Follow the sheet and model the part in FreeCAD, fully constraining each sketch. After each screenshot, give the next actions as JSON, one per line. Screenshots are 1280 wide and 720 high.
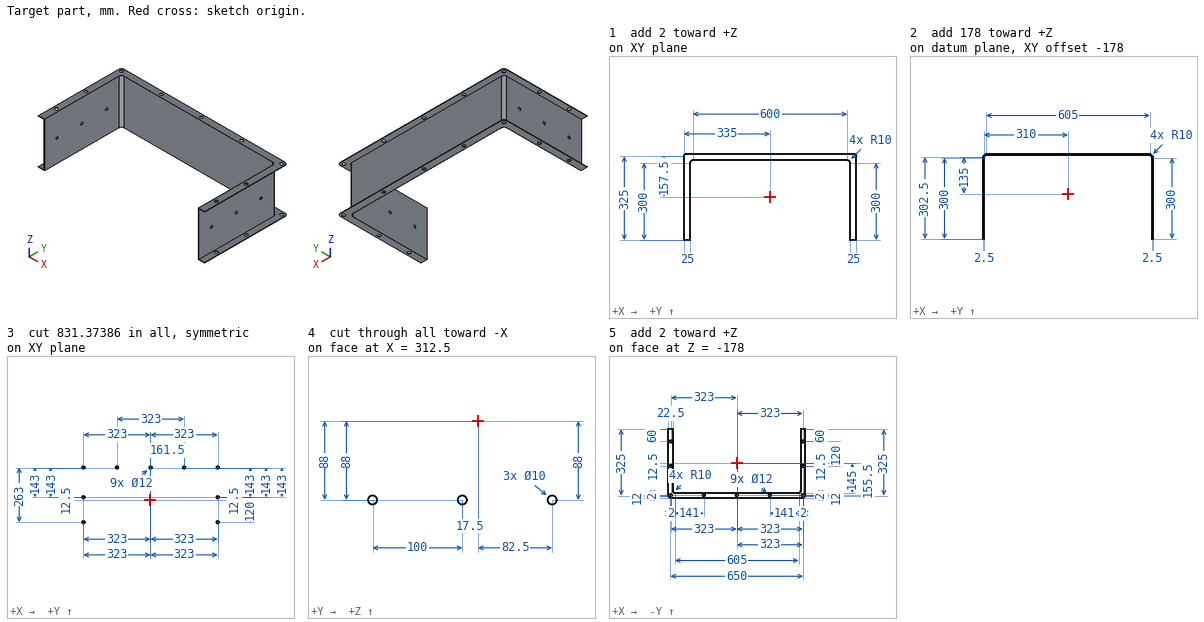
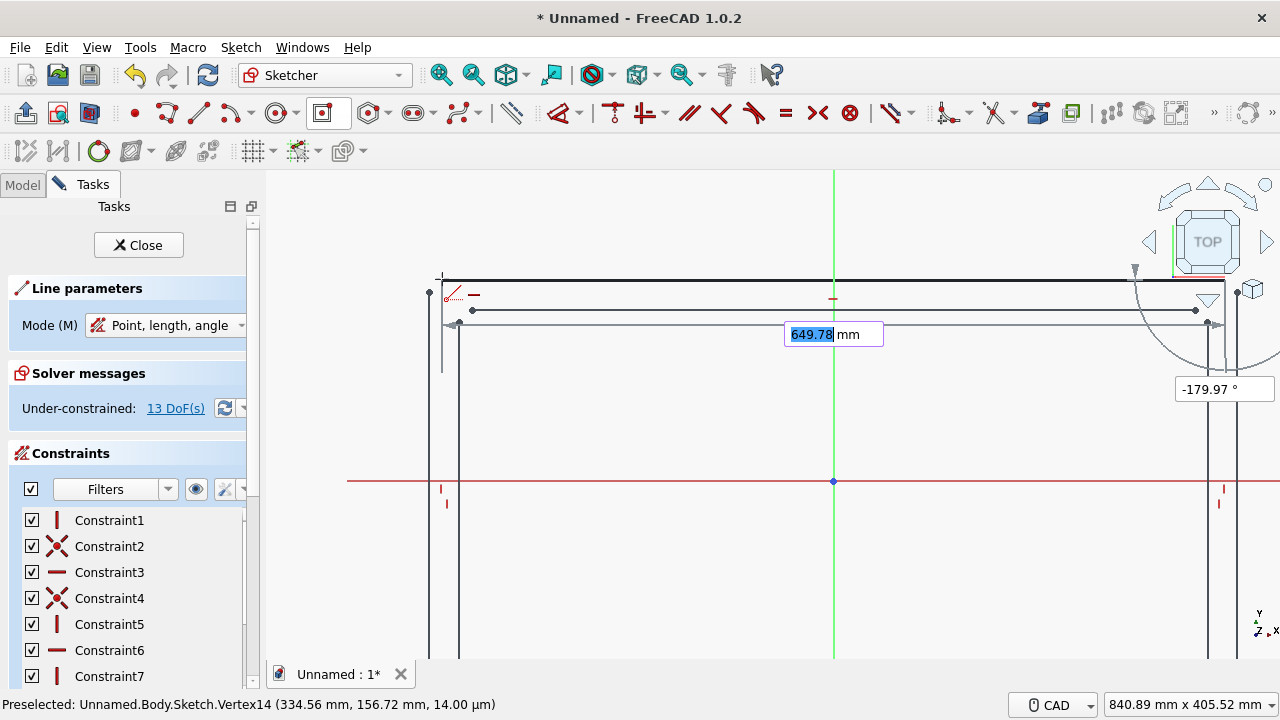
{"action": "left_click", "coordinate": [442, 279]}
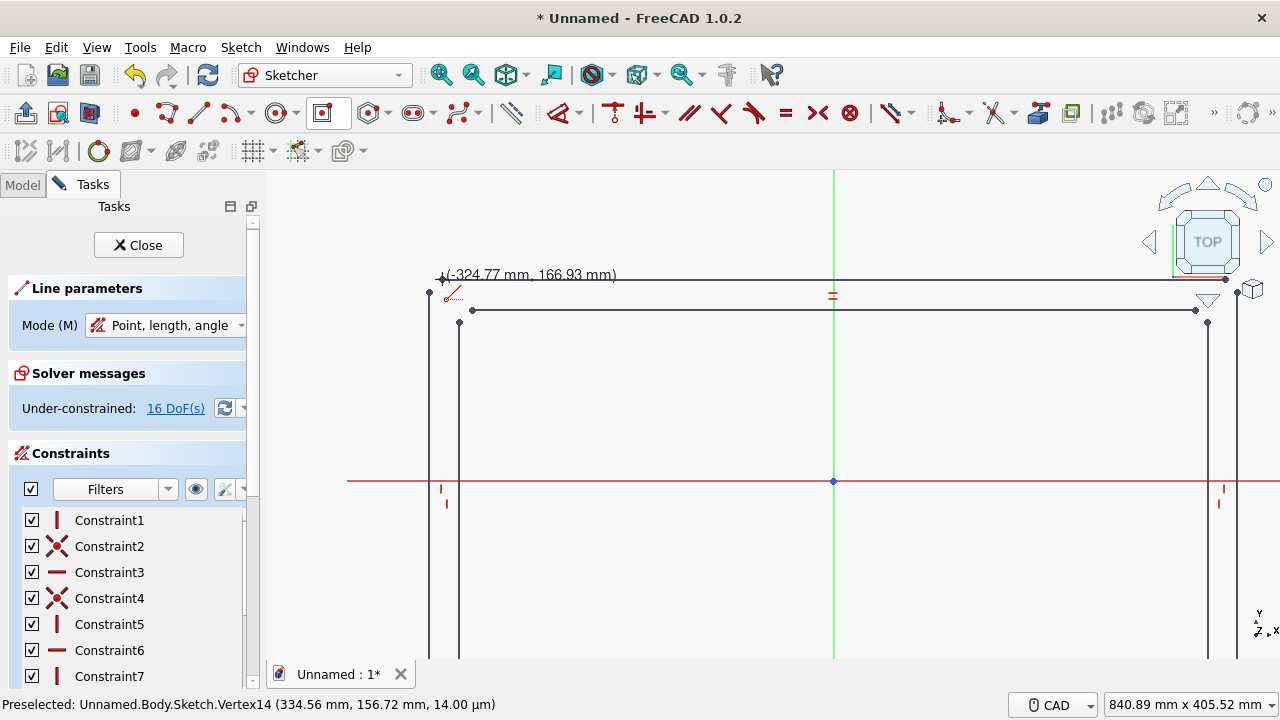
{"action": "left_click", "coordinate": [254, 114]}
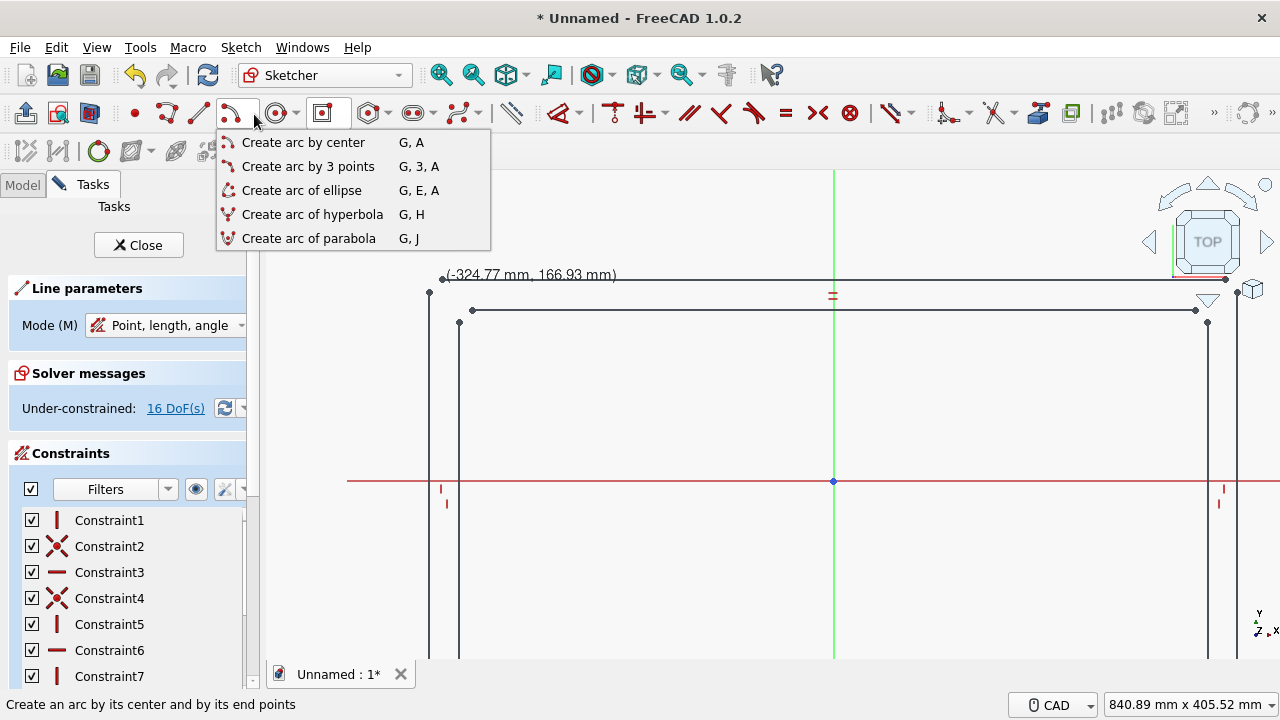
{"action": "left_click", "coordinate": [354, 166]}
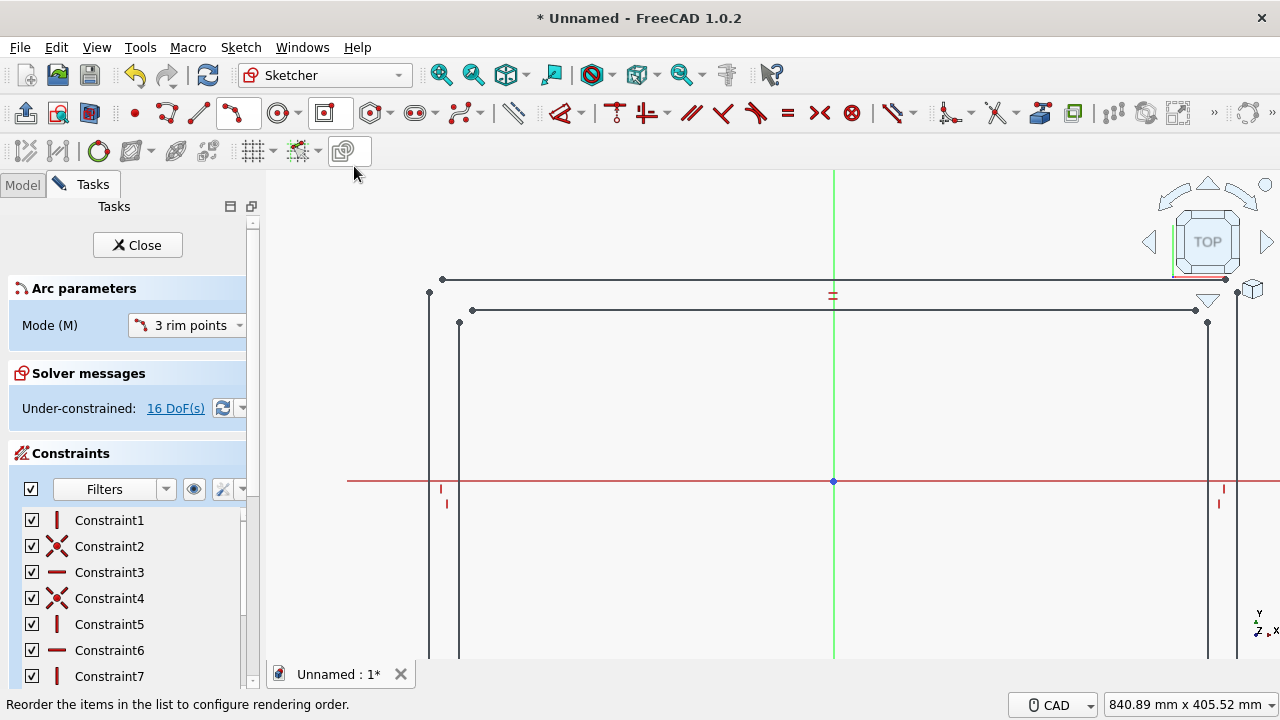
{"action": "left_click", "coordinate": [459, 323]}
{"action": "left_click", "coordinate": [472, 310]}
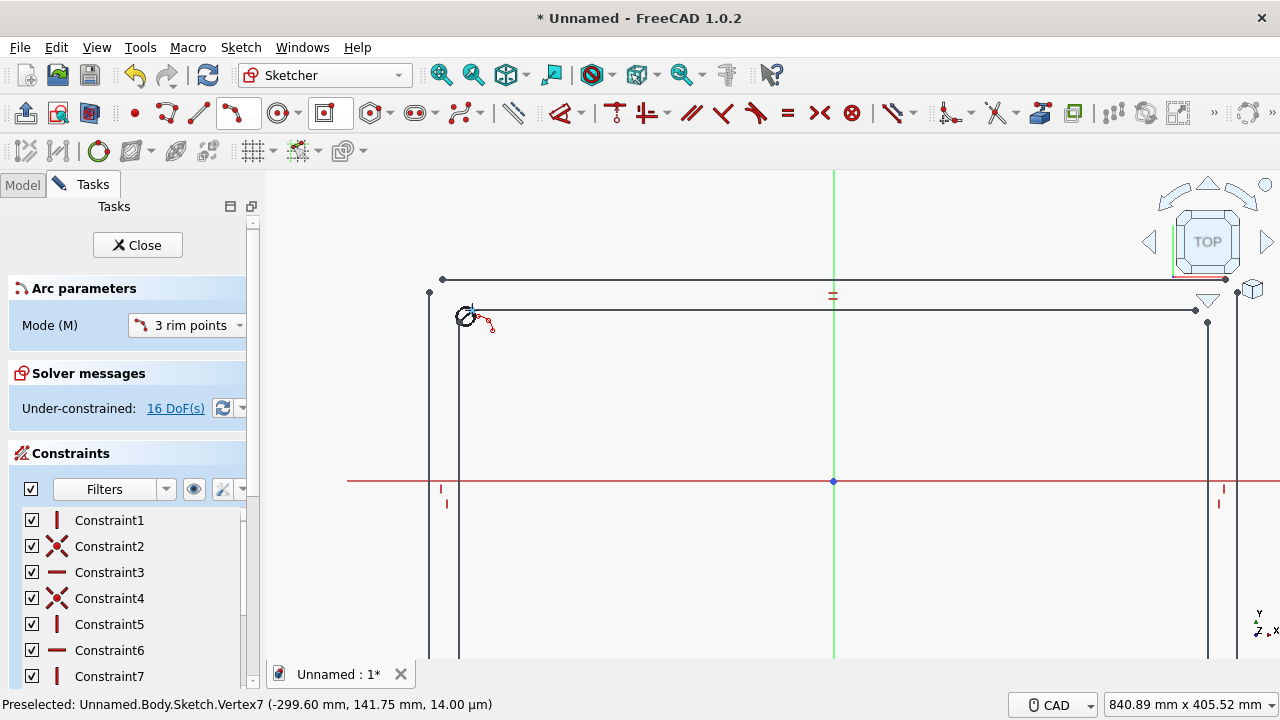
{"action": "scroll", "coordinate": [463, 313], "scroll_direction": "up", "scroll_amount": 8}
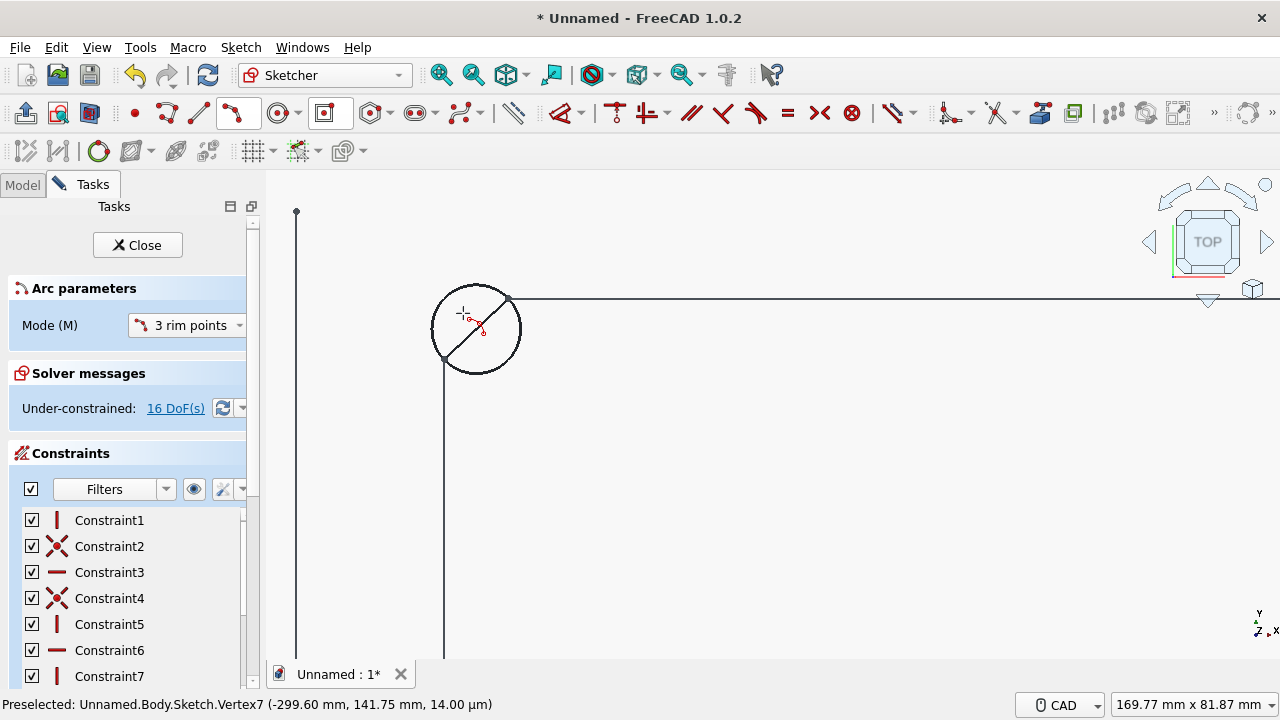
{"action": "left_click", "coordinate": [464, 312]}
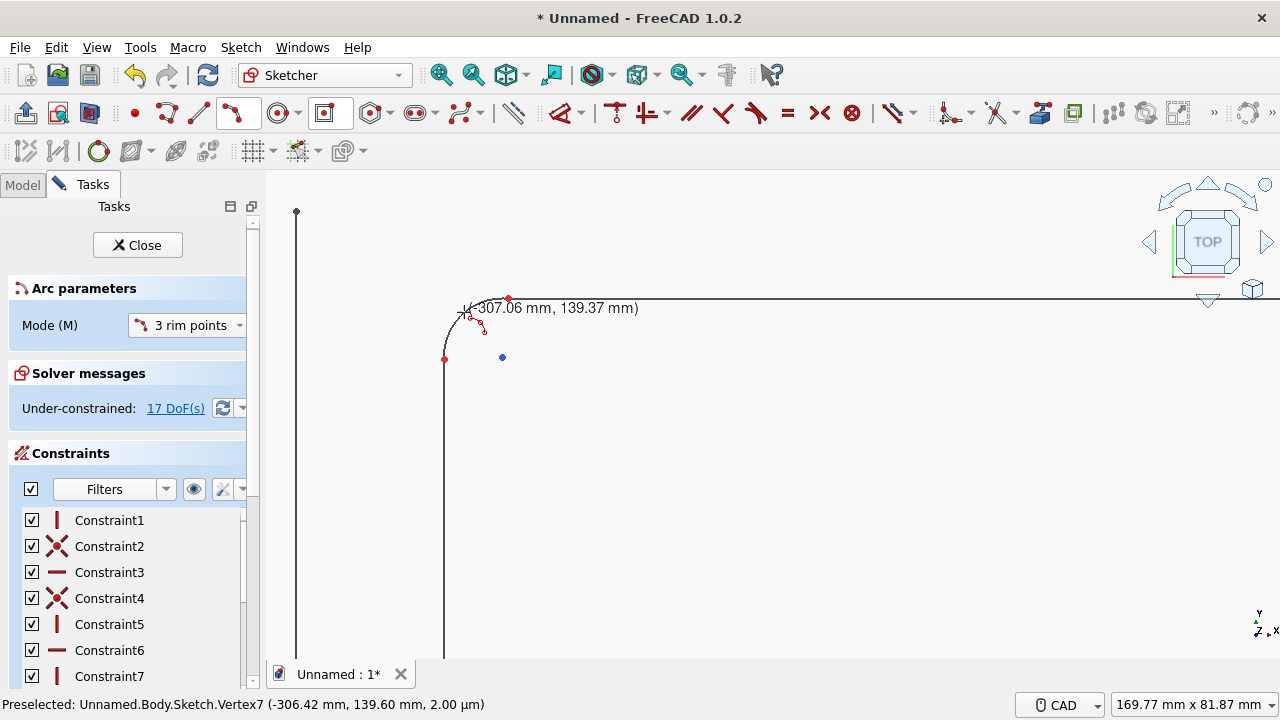
{"action": "scroll", "coordinate": [455, 300], "scroll_direction": "down", "scroll_amount": 10}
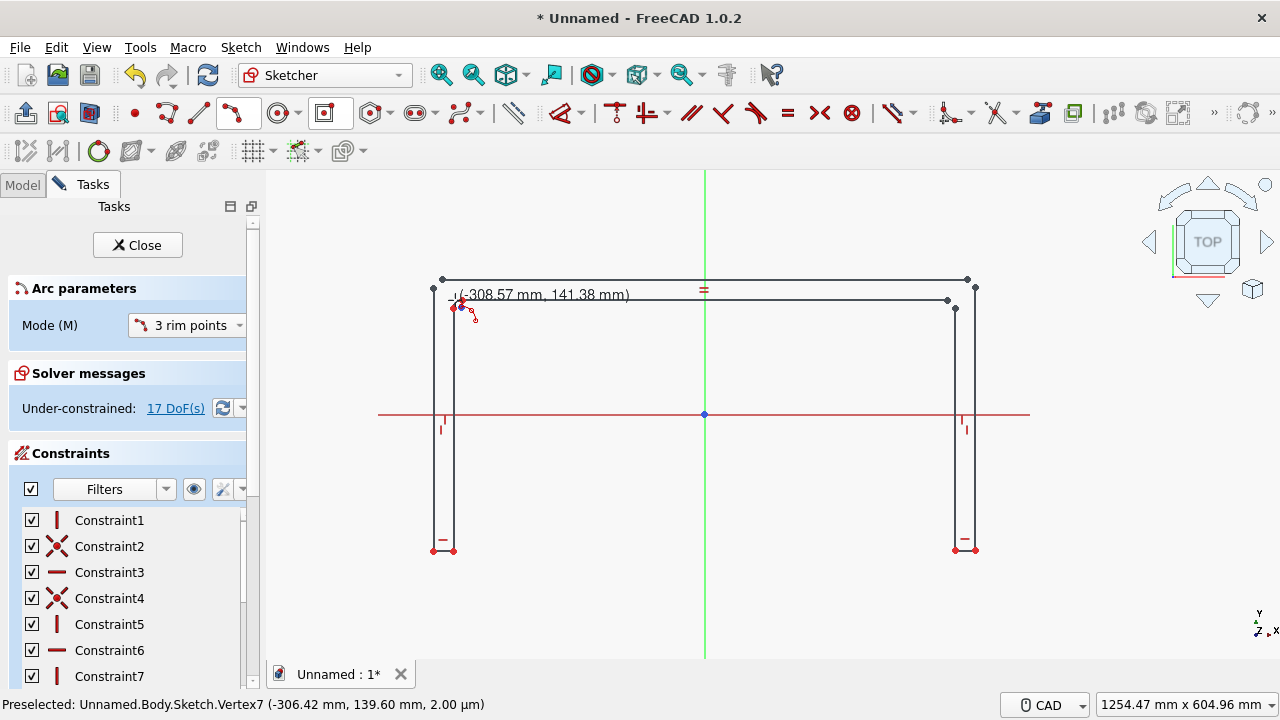
{"action": "scroll", "coordinate": [947, 299], "scroll_direction": "up", "scroll_amount": 2}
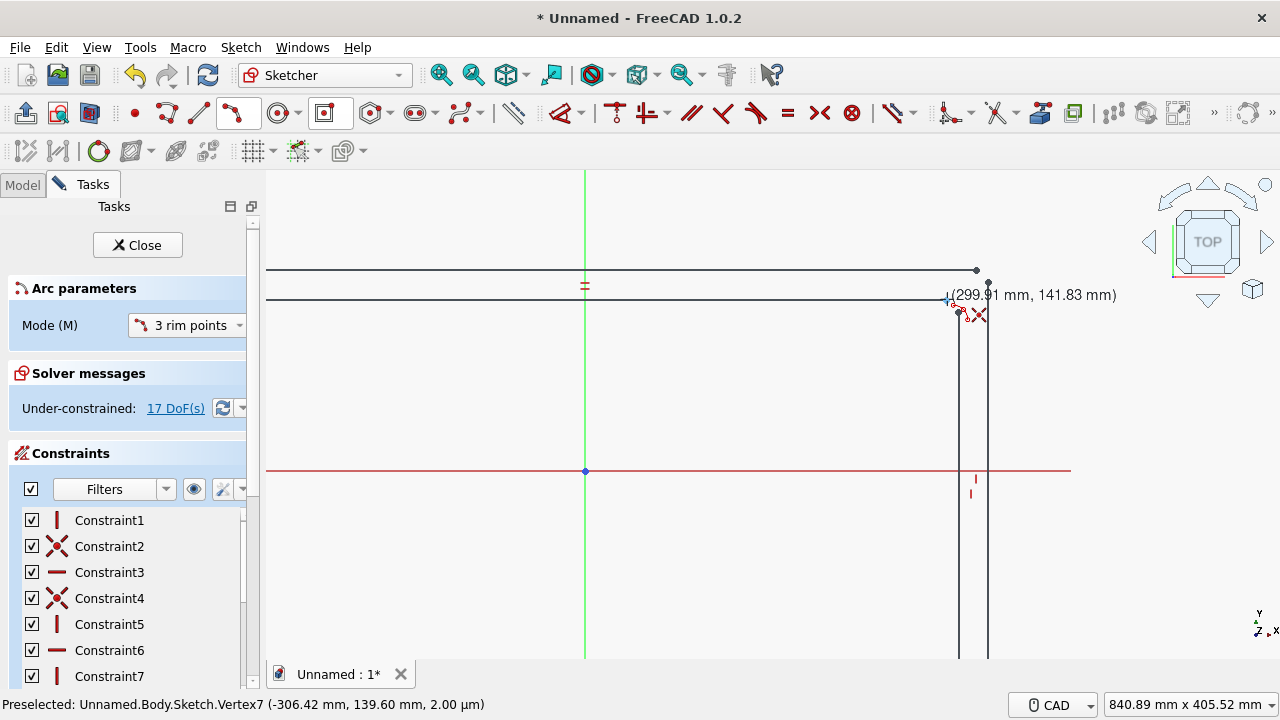
{"action": "left_click", "coordinate": [947, 300]}
{"action": "left_click", "coordinate": [959, 312]}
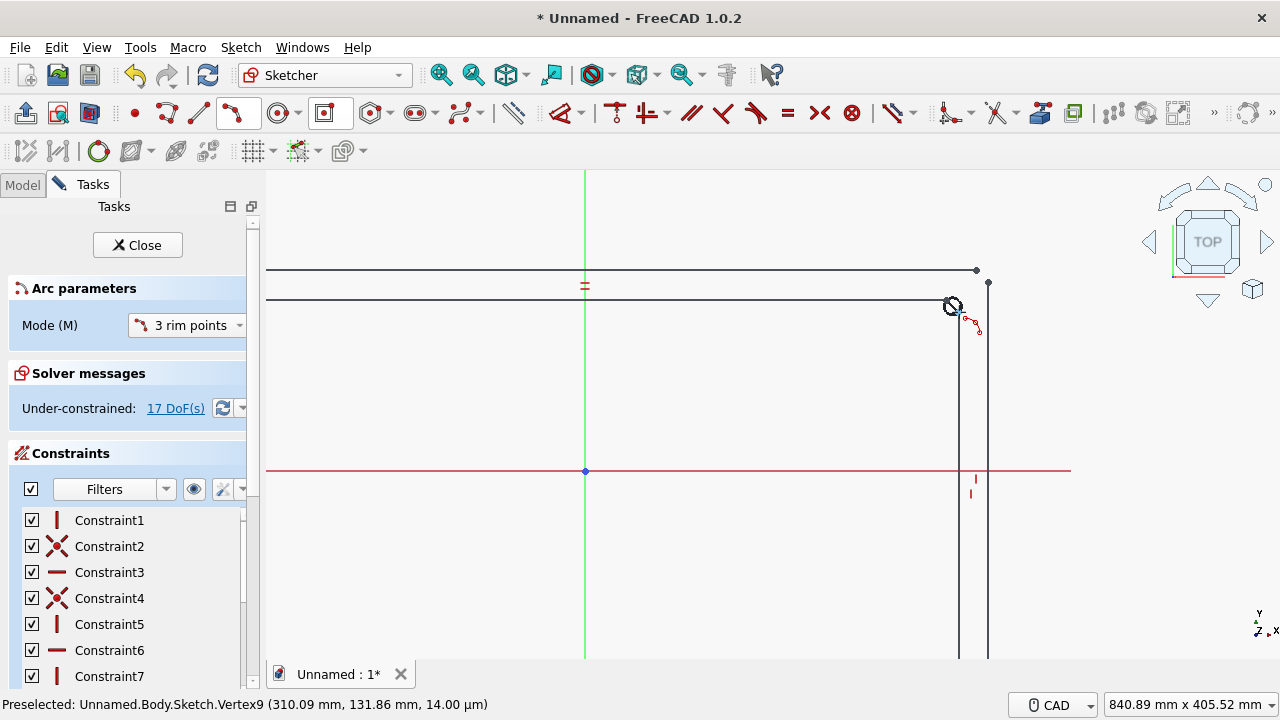
{"action": "scroll", "coordinate": [955, 303], "scroll_direction": "up", "scroll_amount": 8}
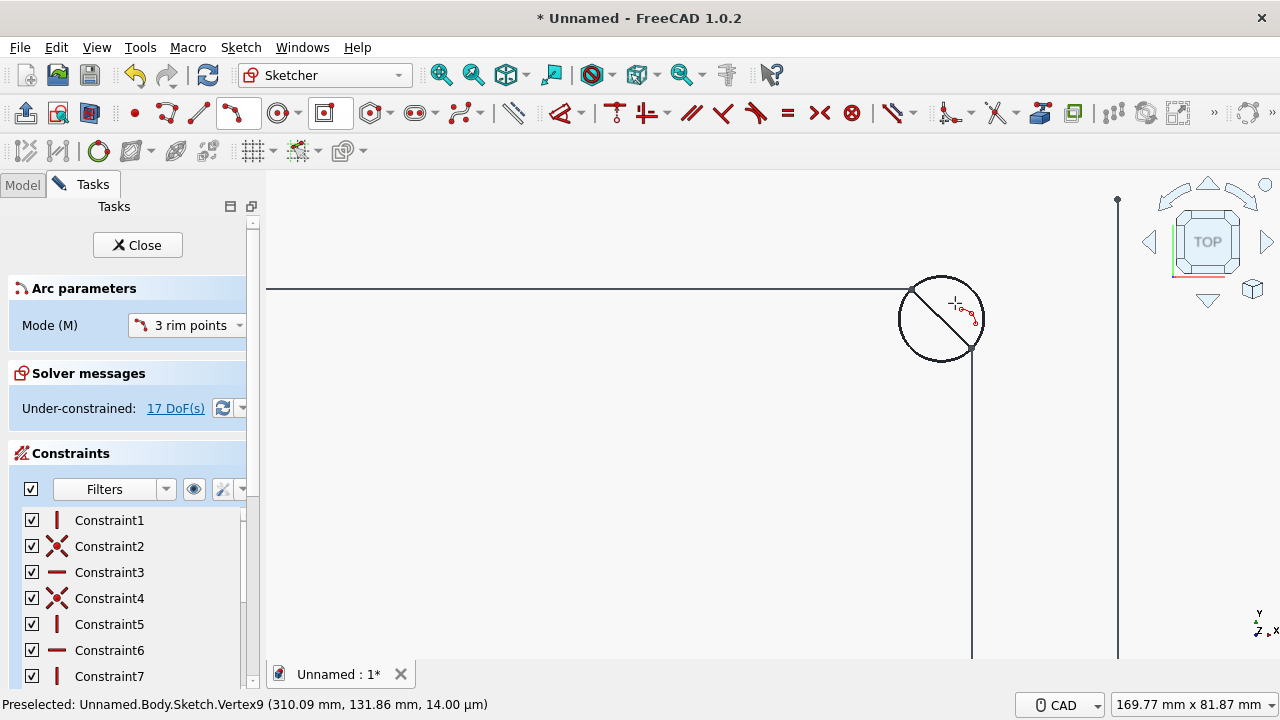
{"action": "left_click", "coordinate": [954, 302]}